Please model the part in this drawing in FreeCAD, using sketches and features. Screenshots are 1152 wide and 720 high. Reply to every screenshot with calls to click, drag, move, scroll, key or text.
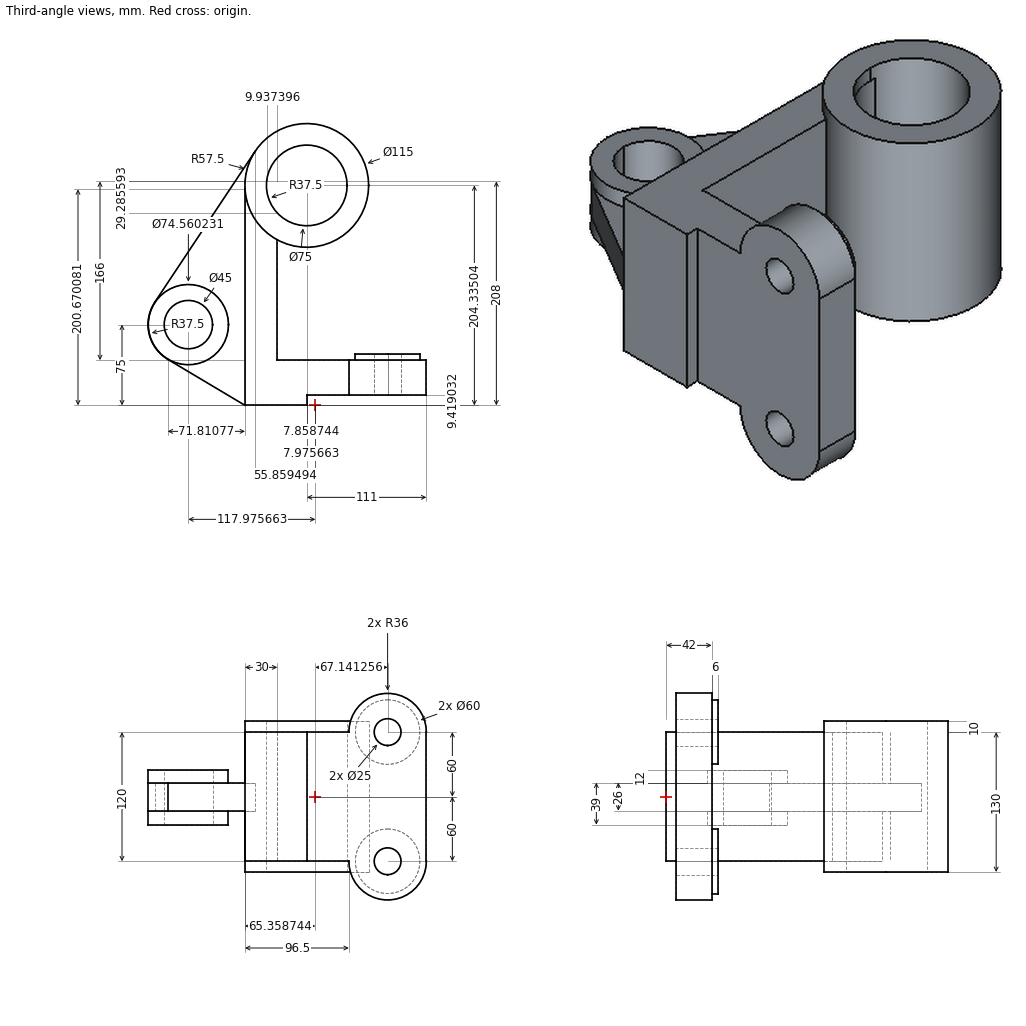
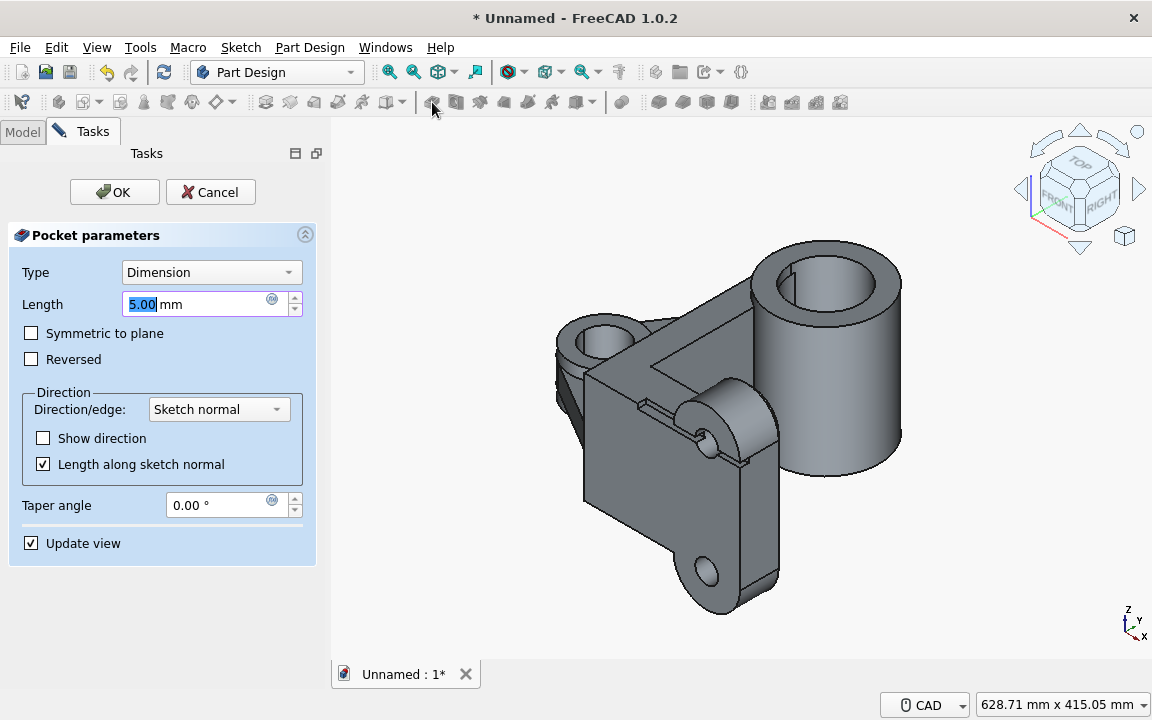
click(212, 272)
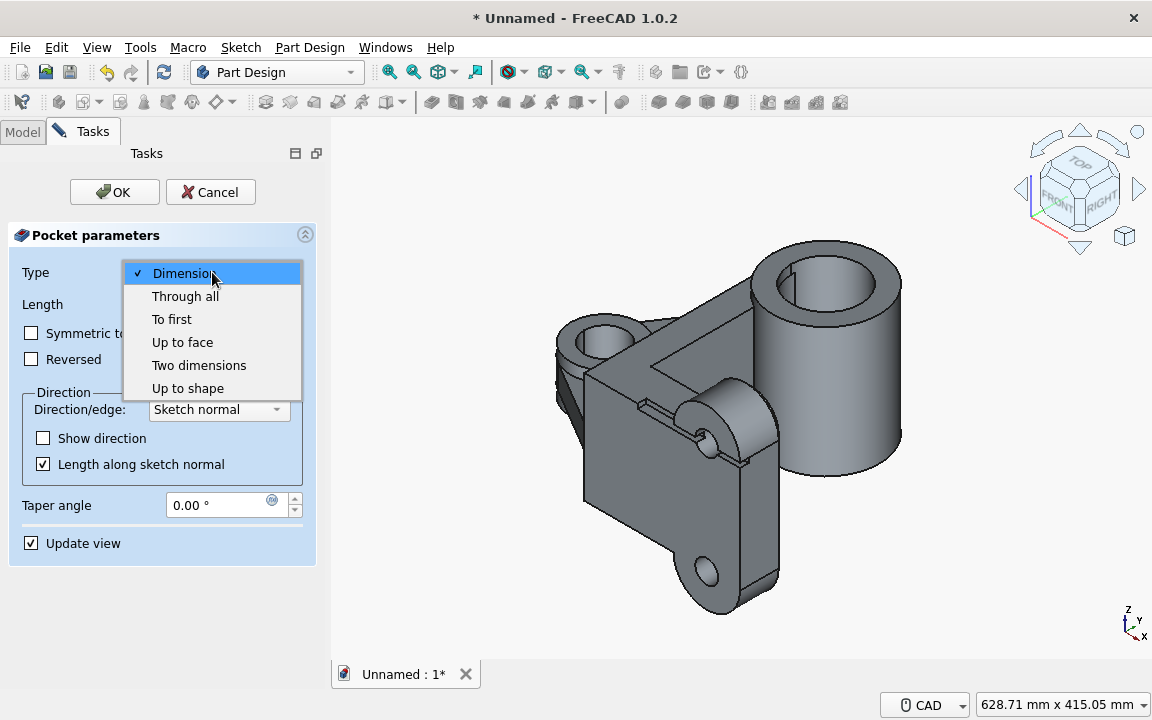
click(212, 366)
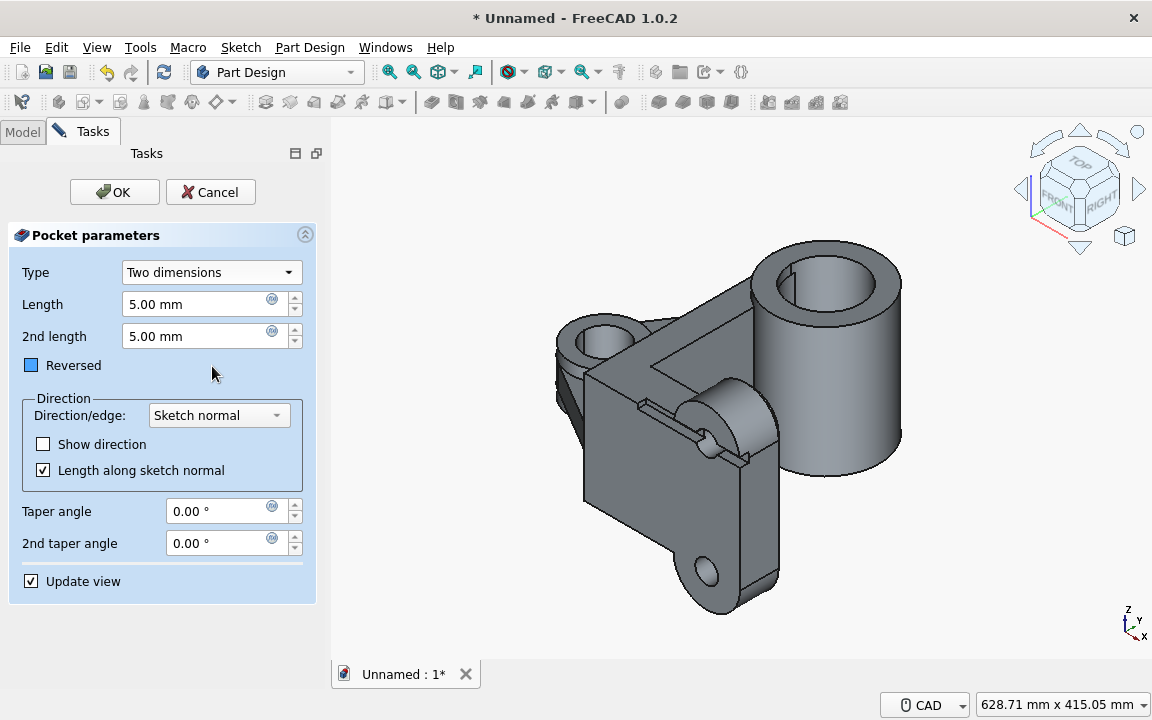
triple_click(204, 304)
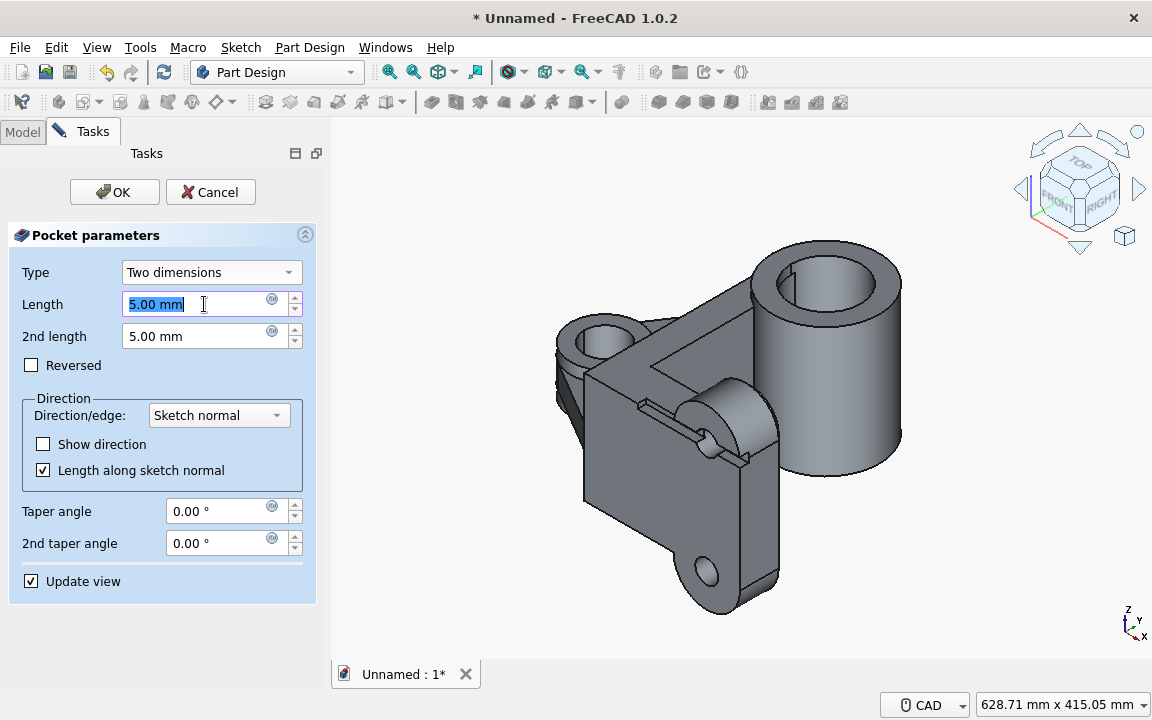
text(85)
key(Tab)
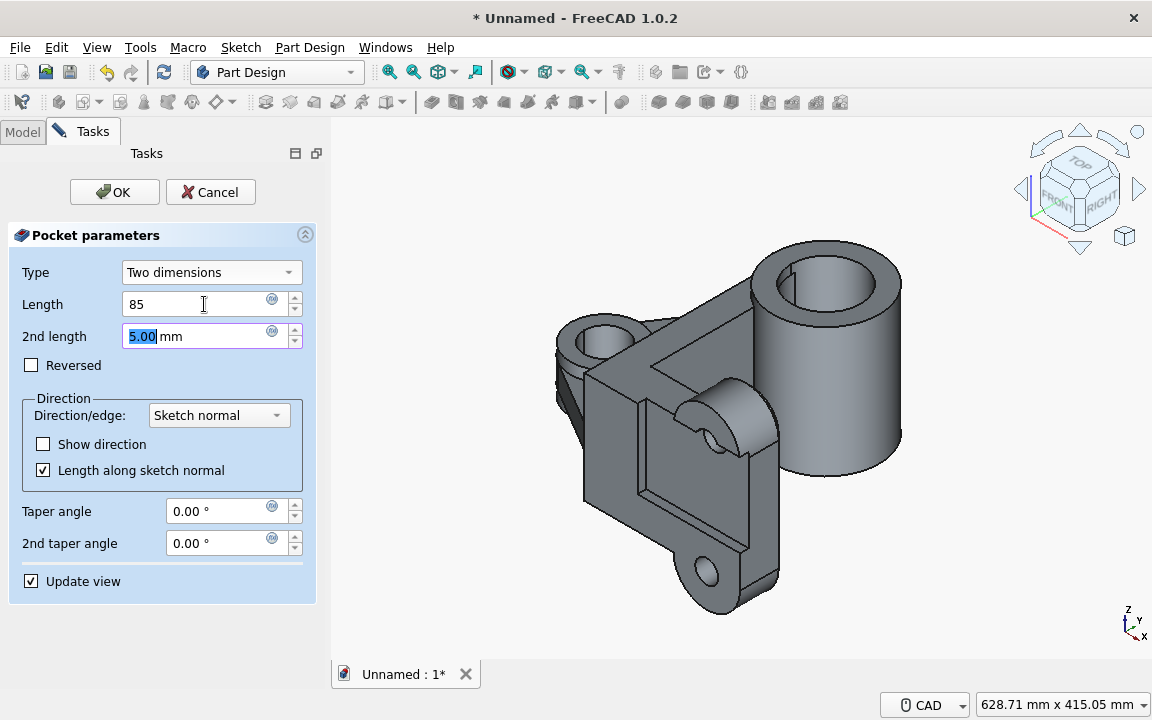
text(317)
key(Tab)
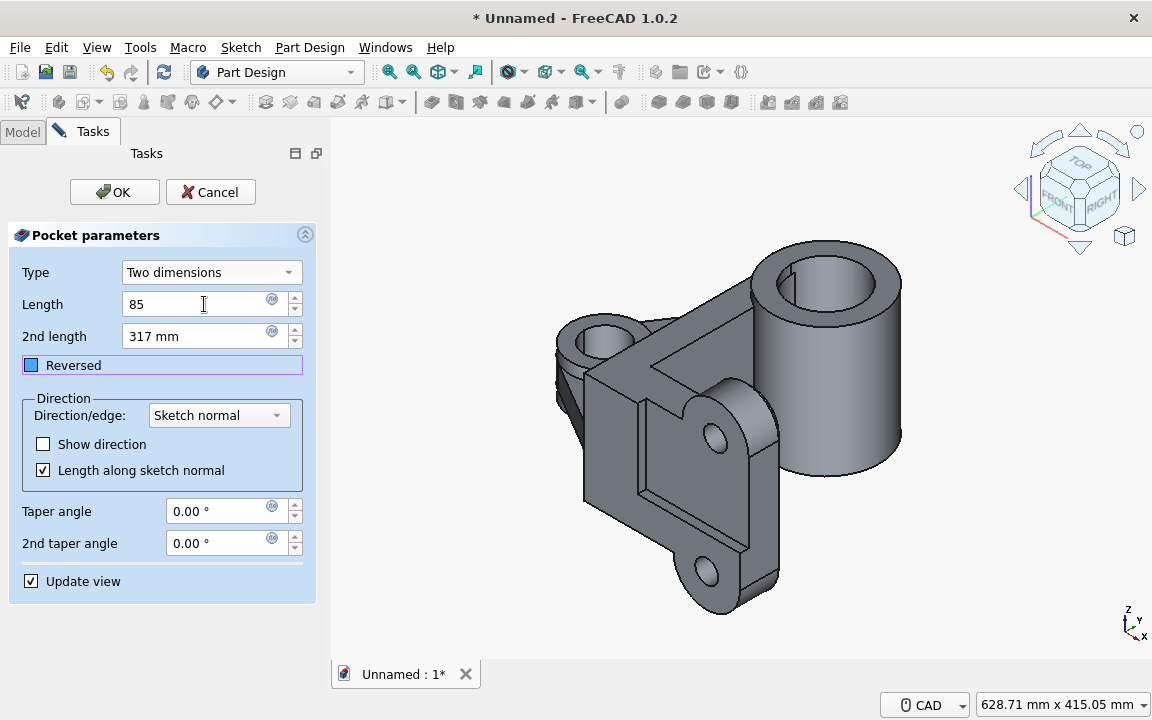
click(30, 365)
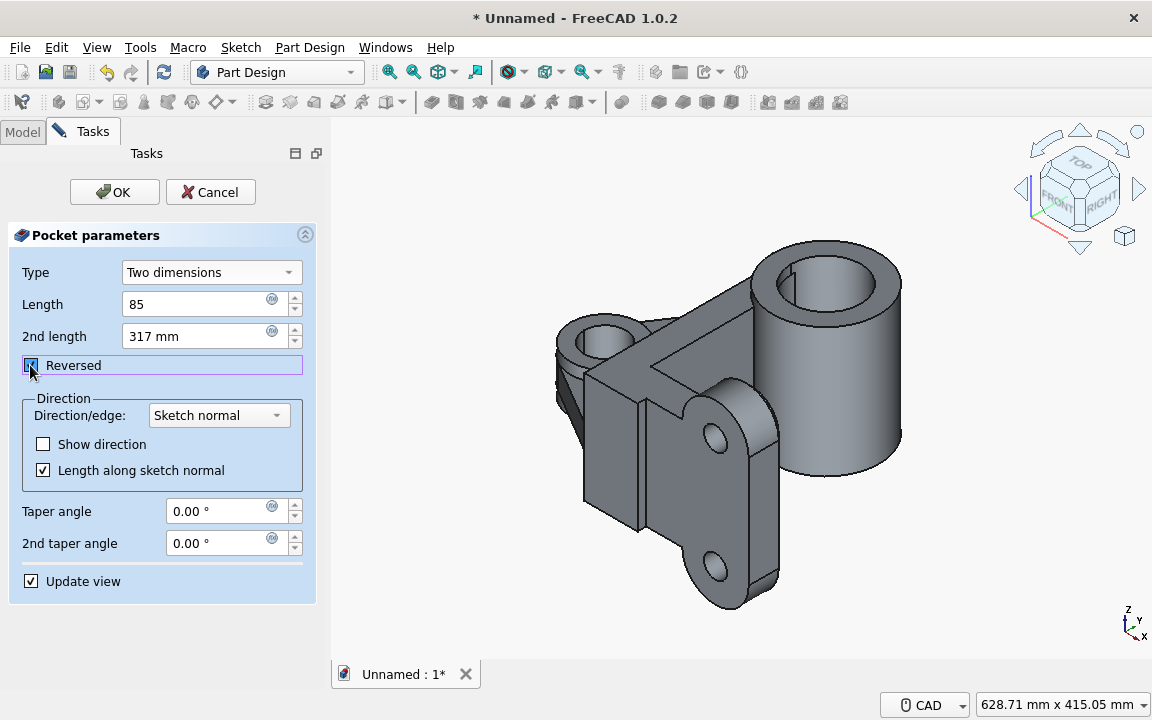
click(115, 192)